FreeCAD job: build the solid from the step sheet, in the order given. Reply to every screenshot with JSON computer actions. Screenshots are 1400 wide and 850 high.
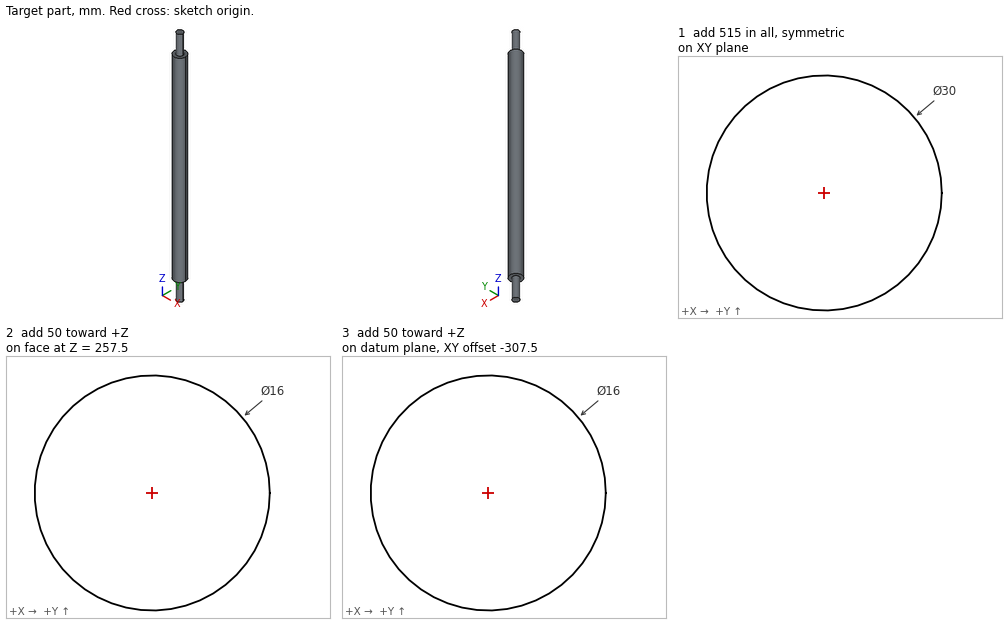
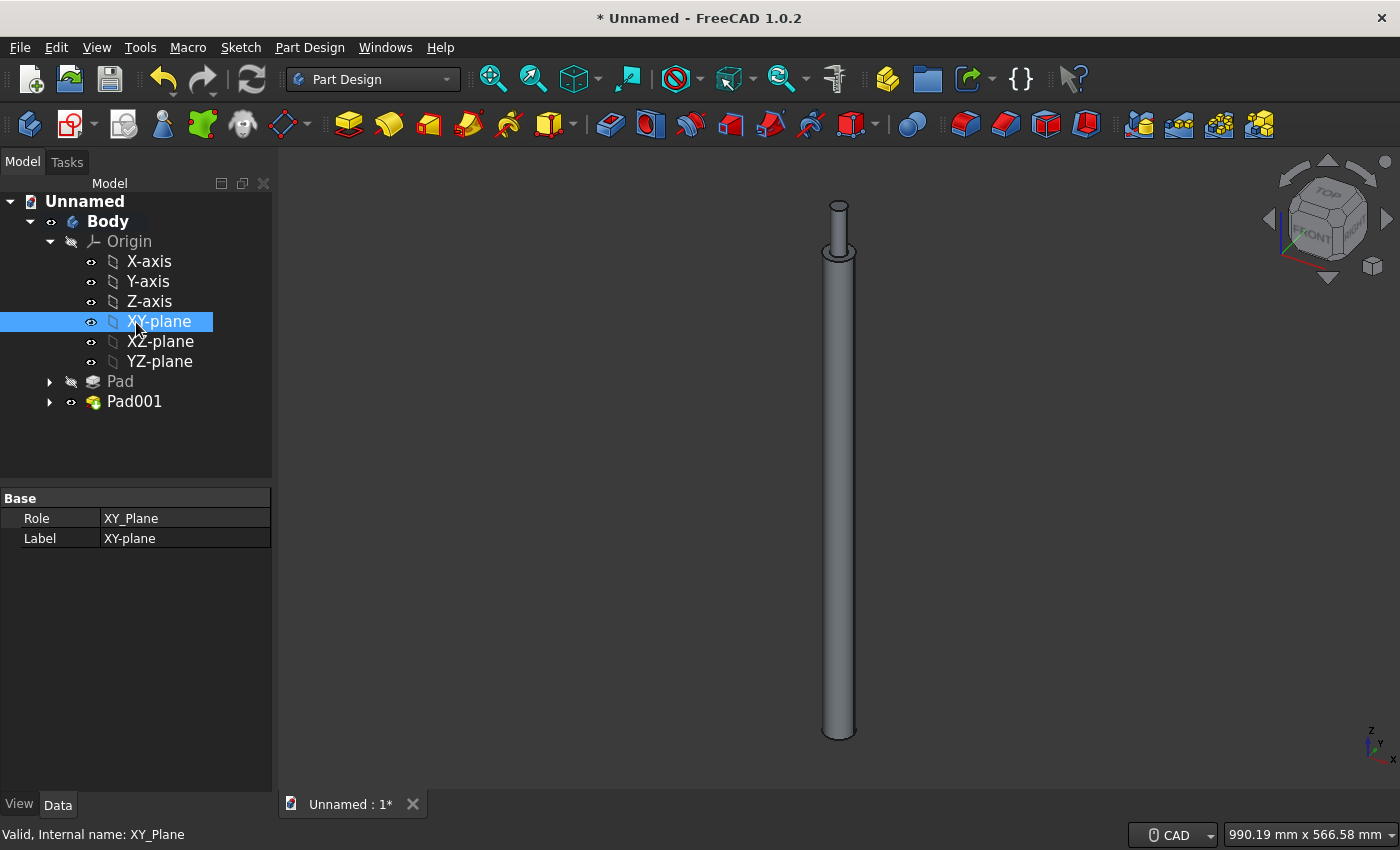
{"action": "left_click", "coordinate": [284, 124]}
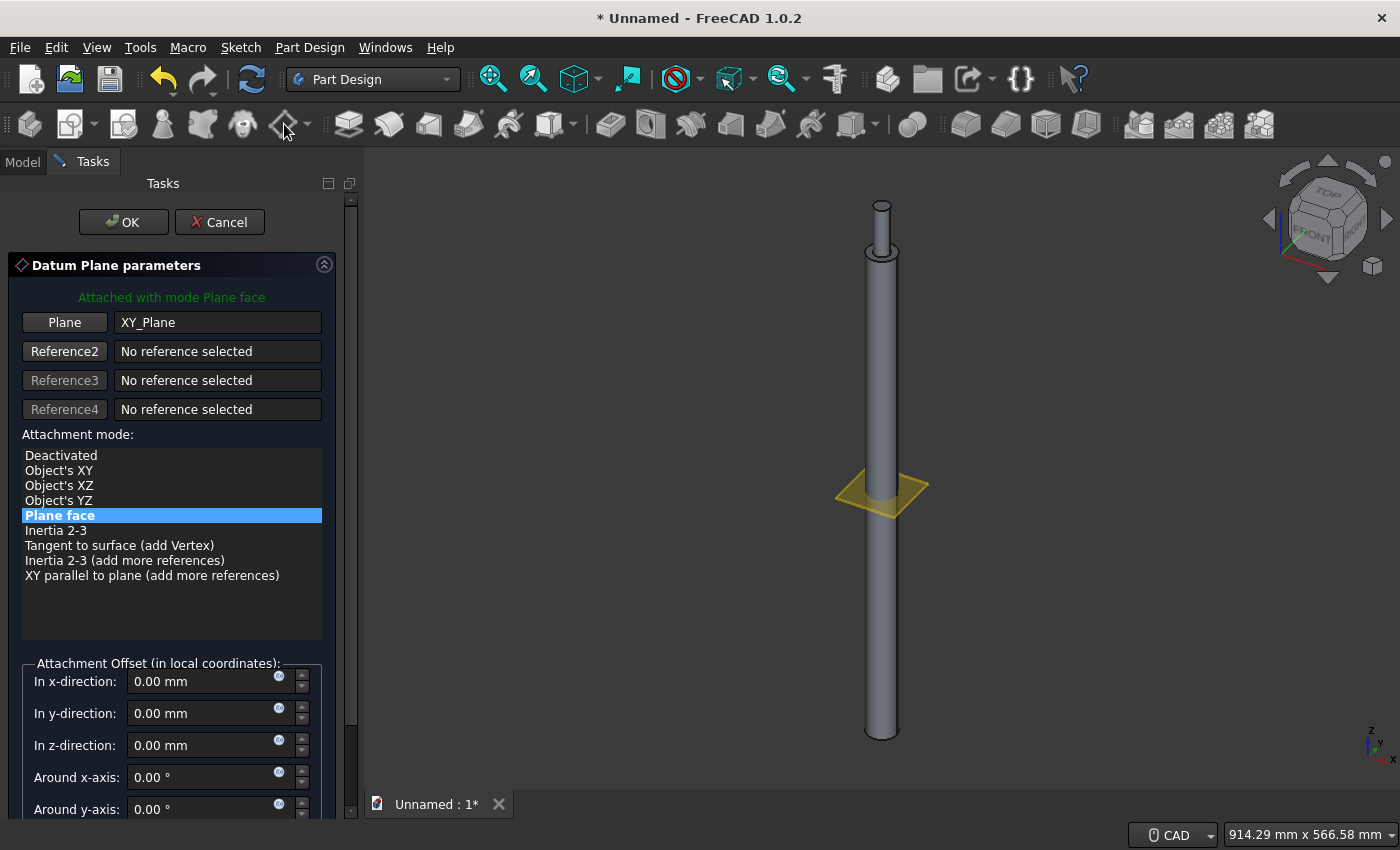
{"action": "triple_click", "coordinate": [210, 745]}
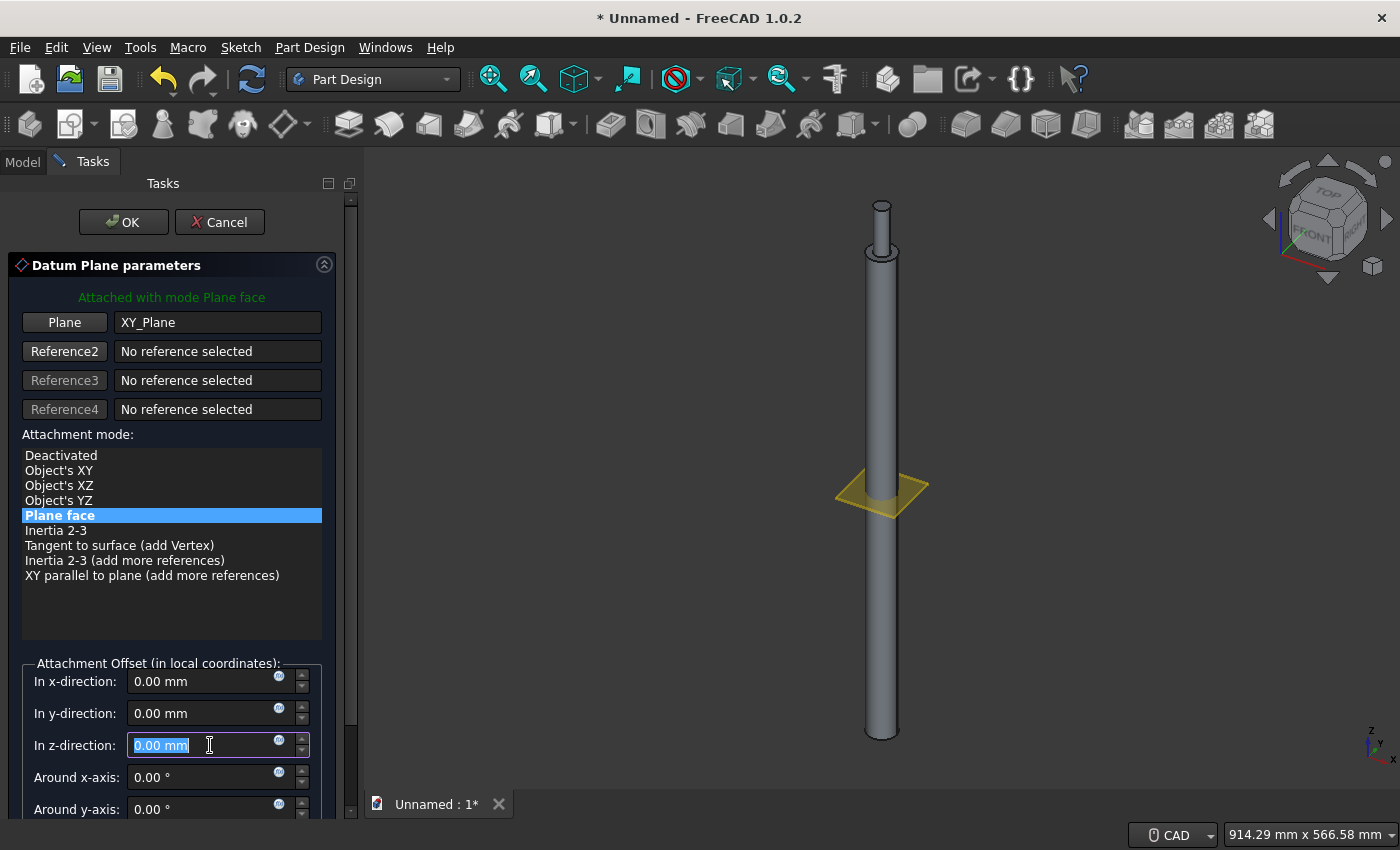
{"action": "type", "text": "-307.5"}
{"action": "key", "text": "Tab"}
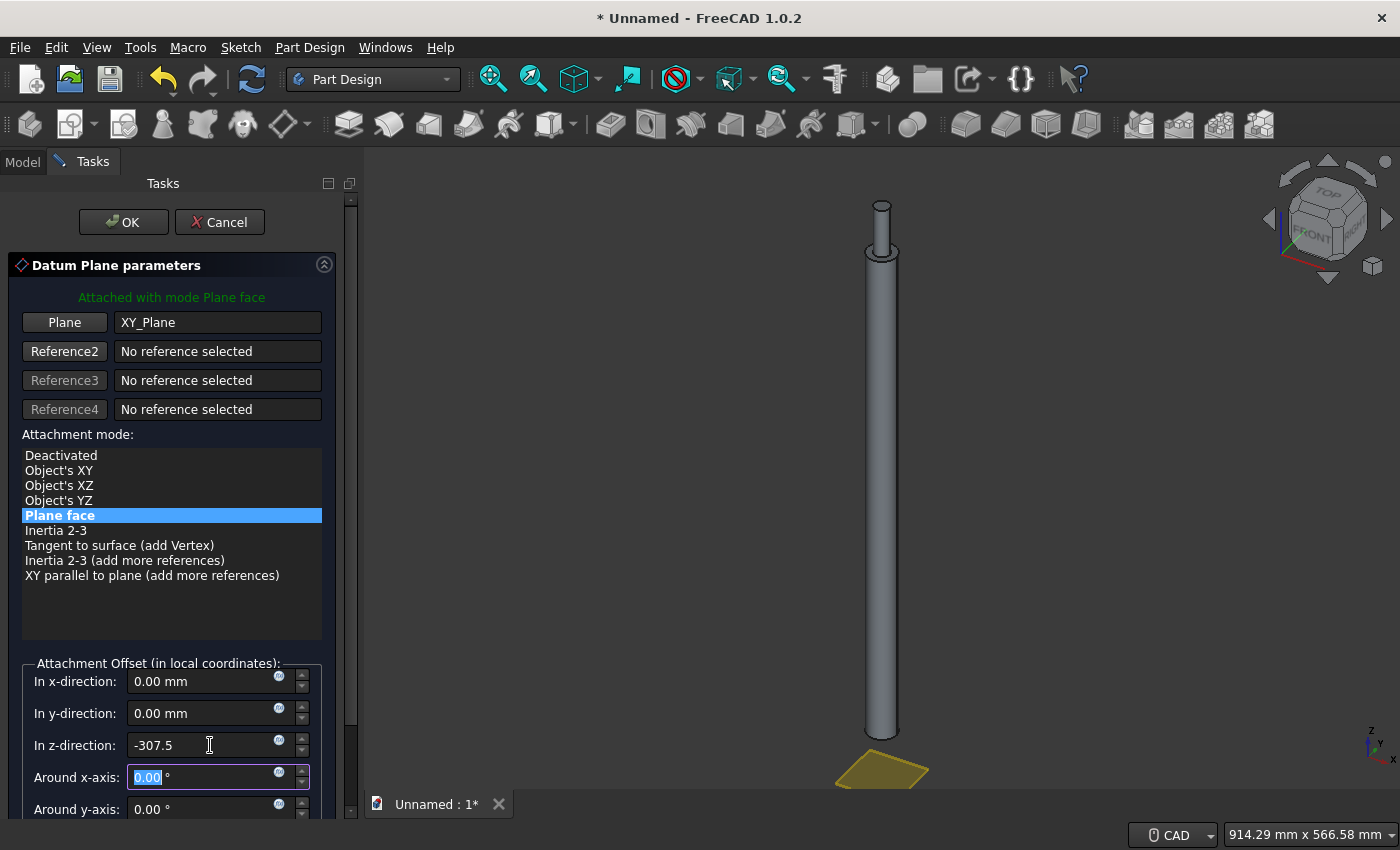
{"action": "left_click", "coordinate": [124, 222]}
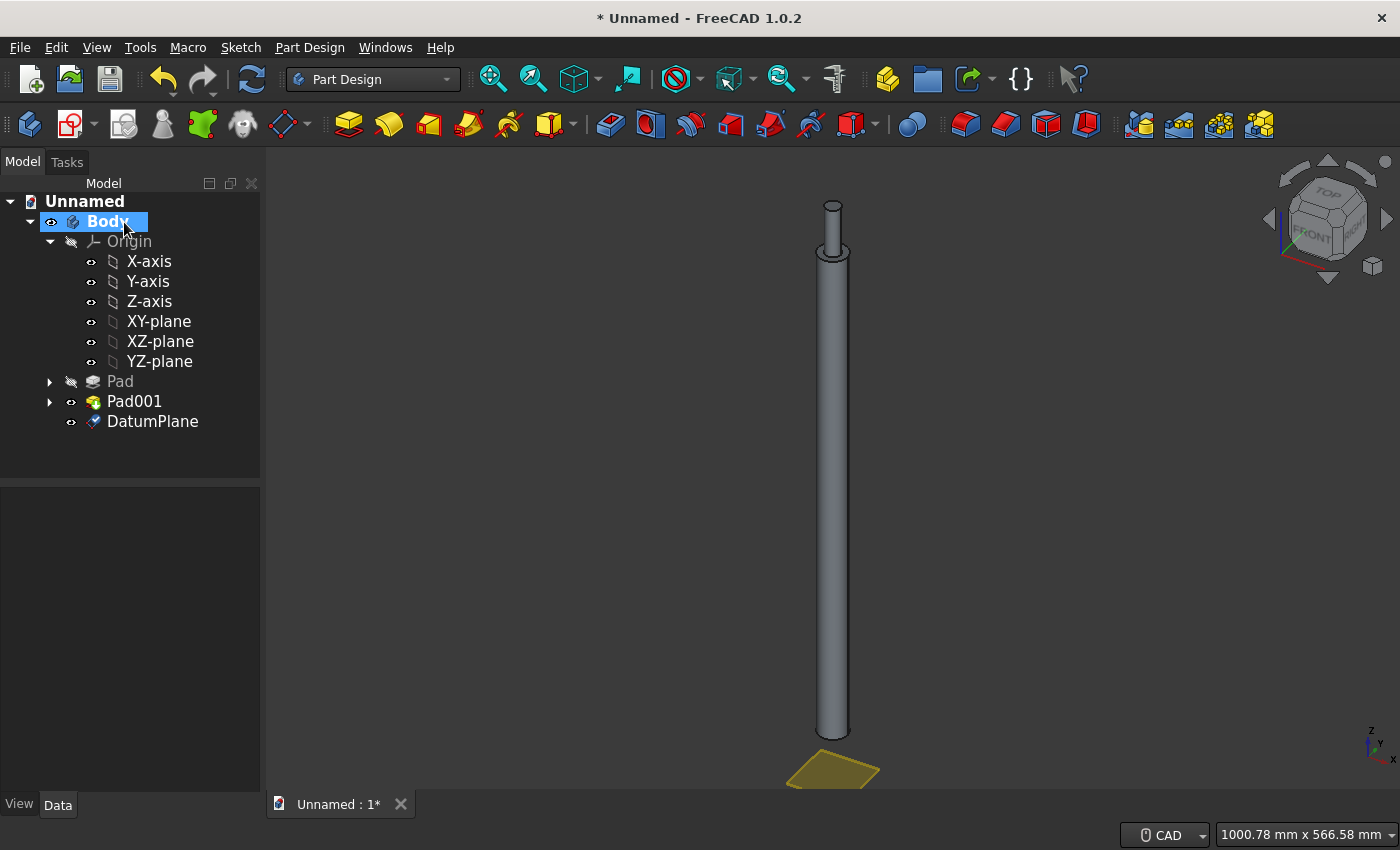
{"action": "left_click", "coordinate": [116, 422]}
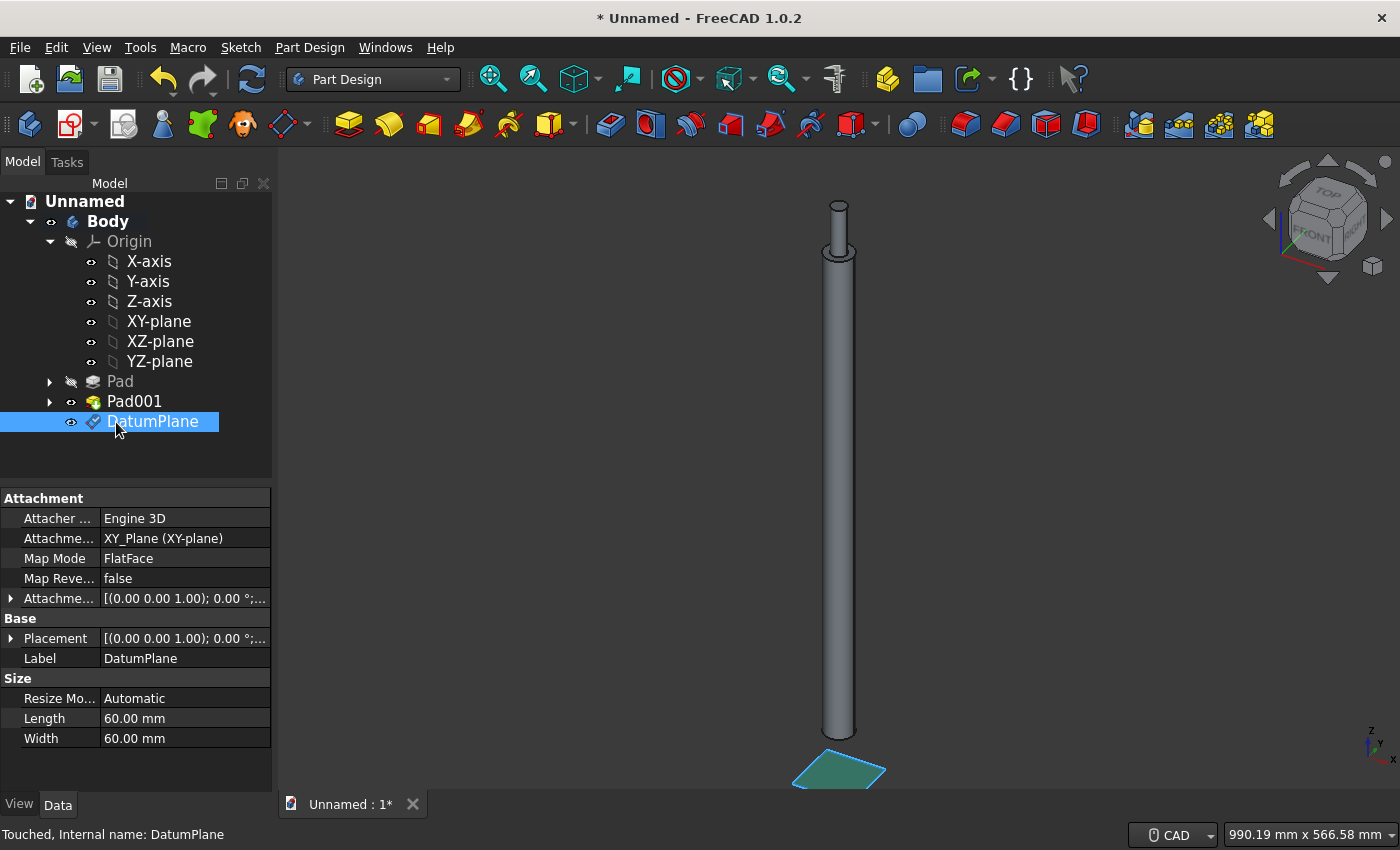
{"action": "left_click", "coordinate": [70, 124]}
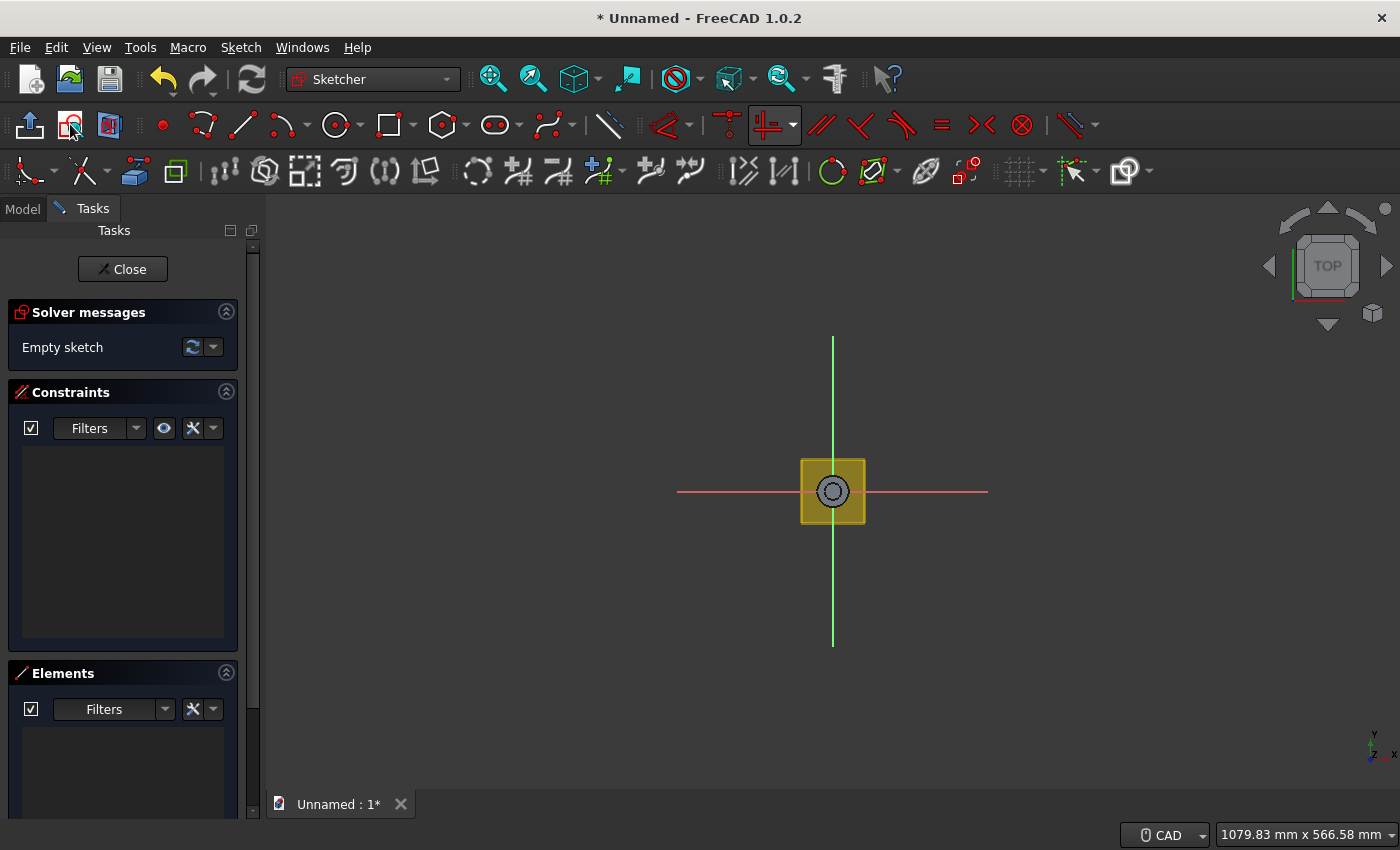
{"action": "key", "text": "q s"}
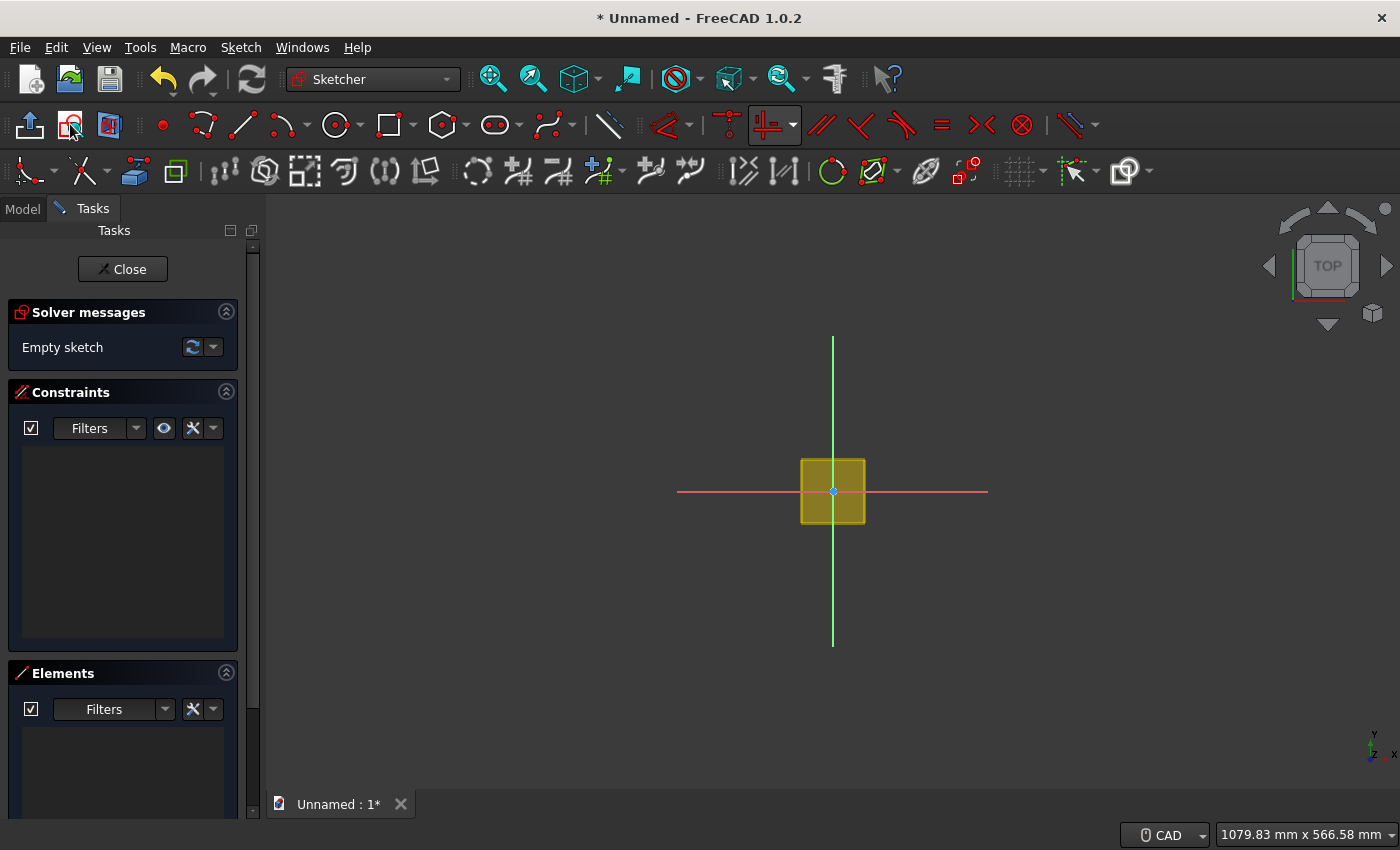
{"action": "scroll", "coordinate": [837, 492], "scroll_direction": "up", "scroll_amount": 15}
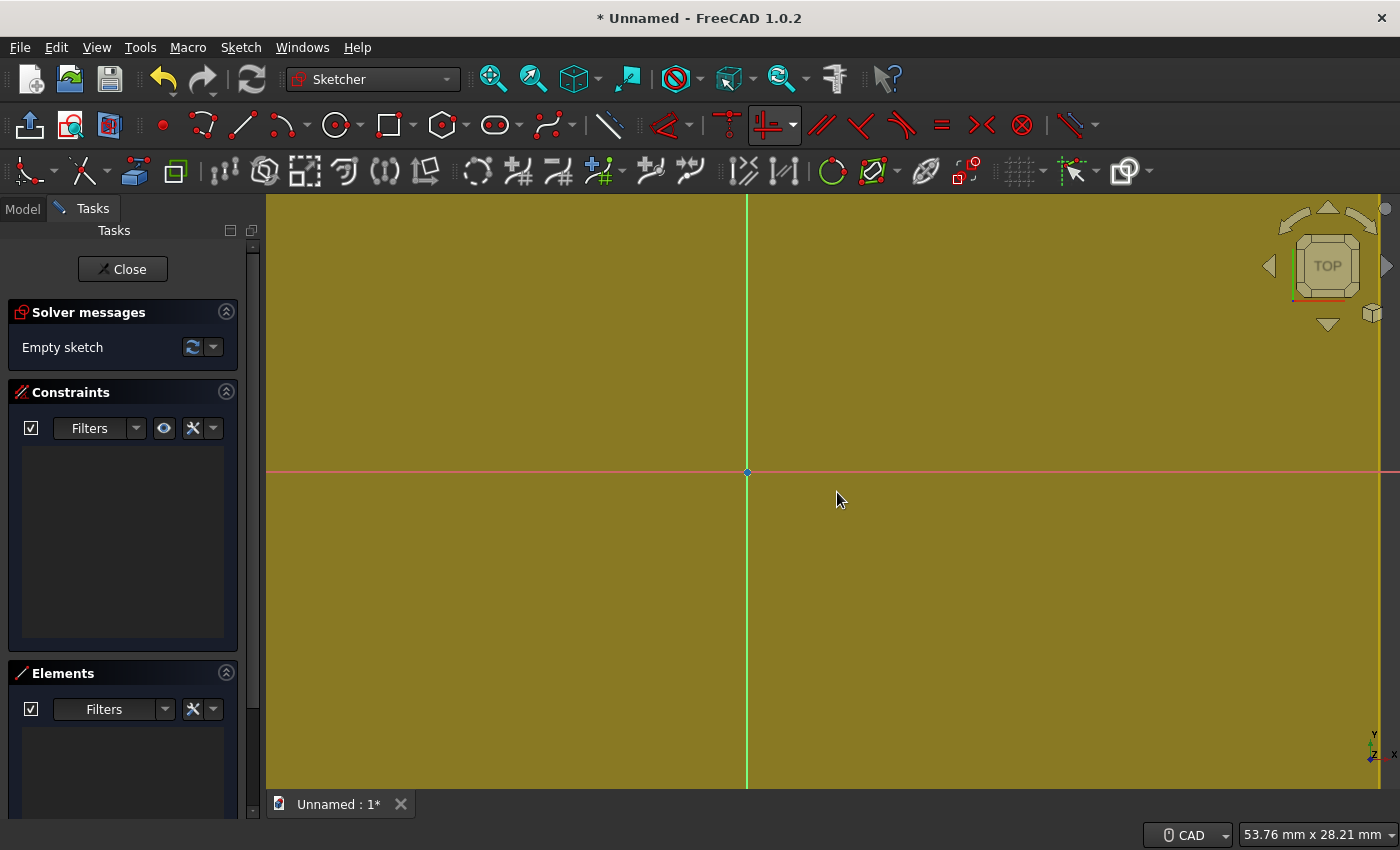
{"action": "key", "text": "g c"}